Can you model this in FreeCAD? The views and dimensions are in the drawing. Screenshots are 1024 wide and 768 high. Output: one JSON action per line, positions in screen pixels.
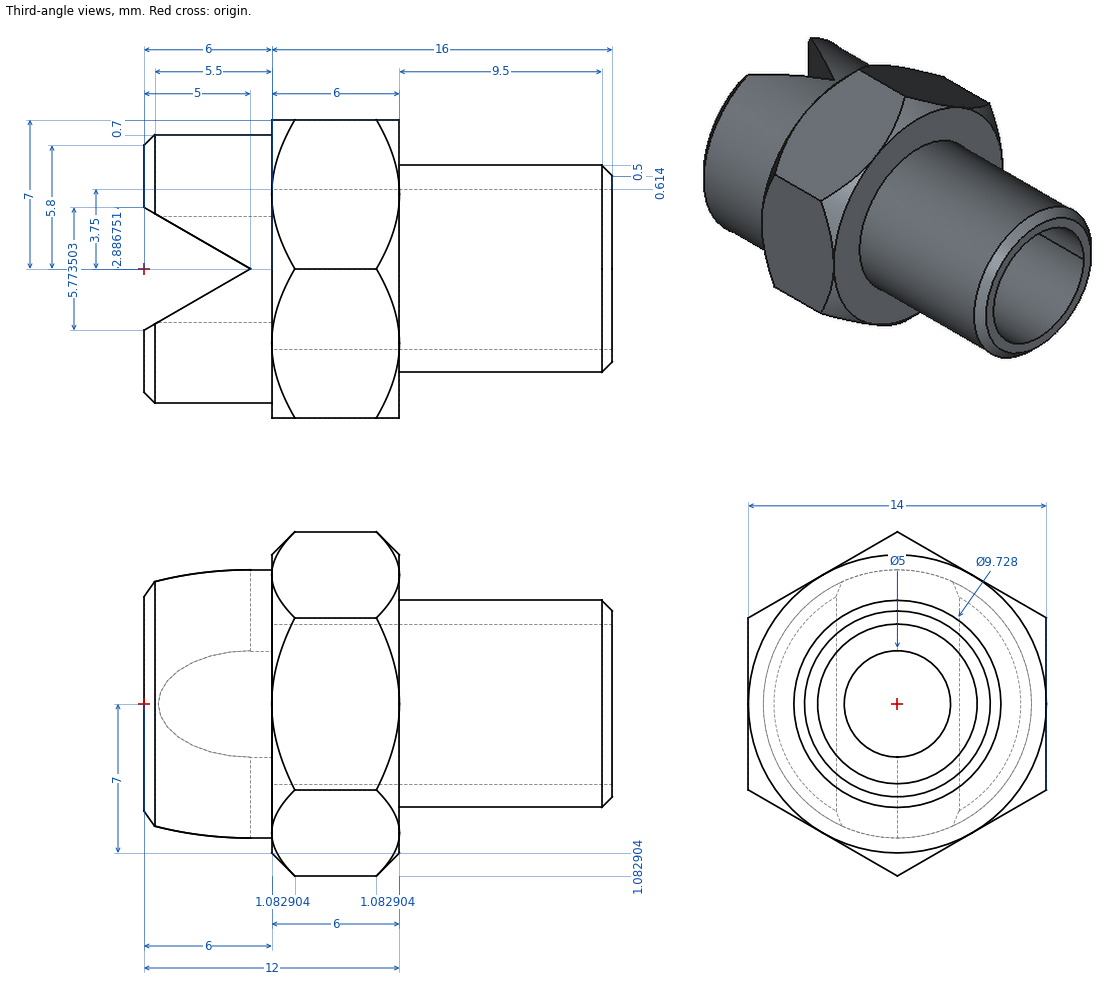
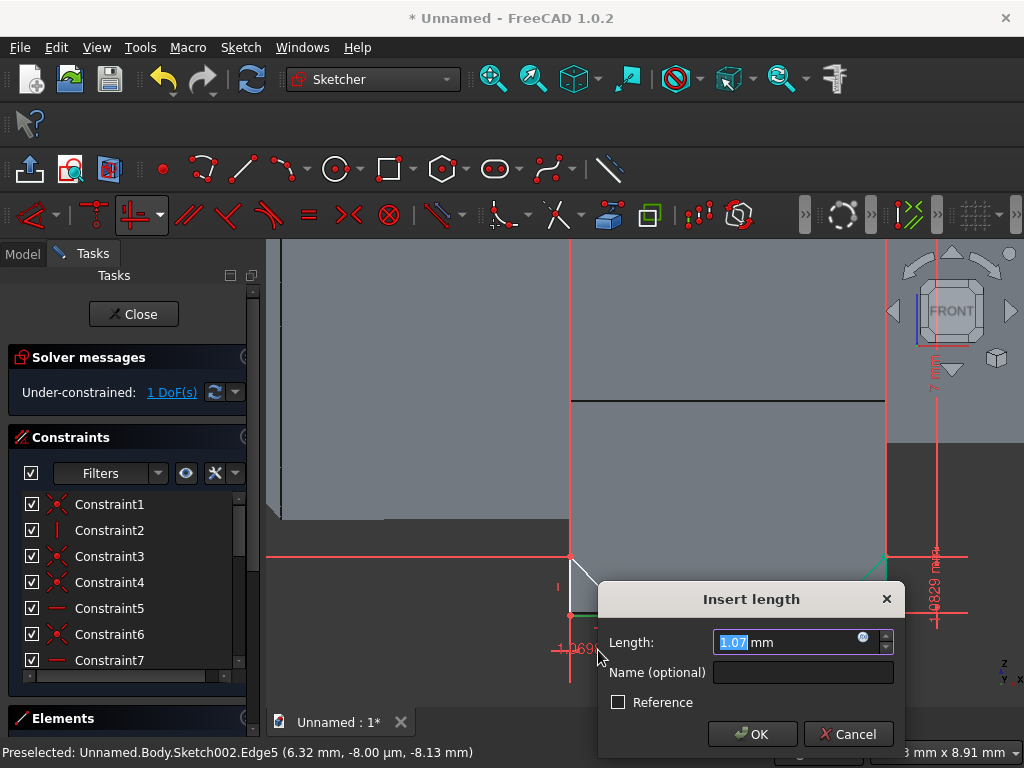
{"action": "type", "text": "1.082904"}
{"action": "key", "text": "Return"}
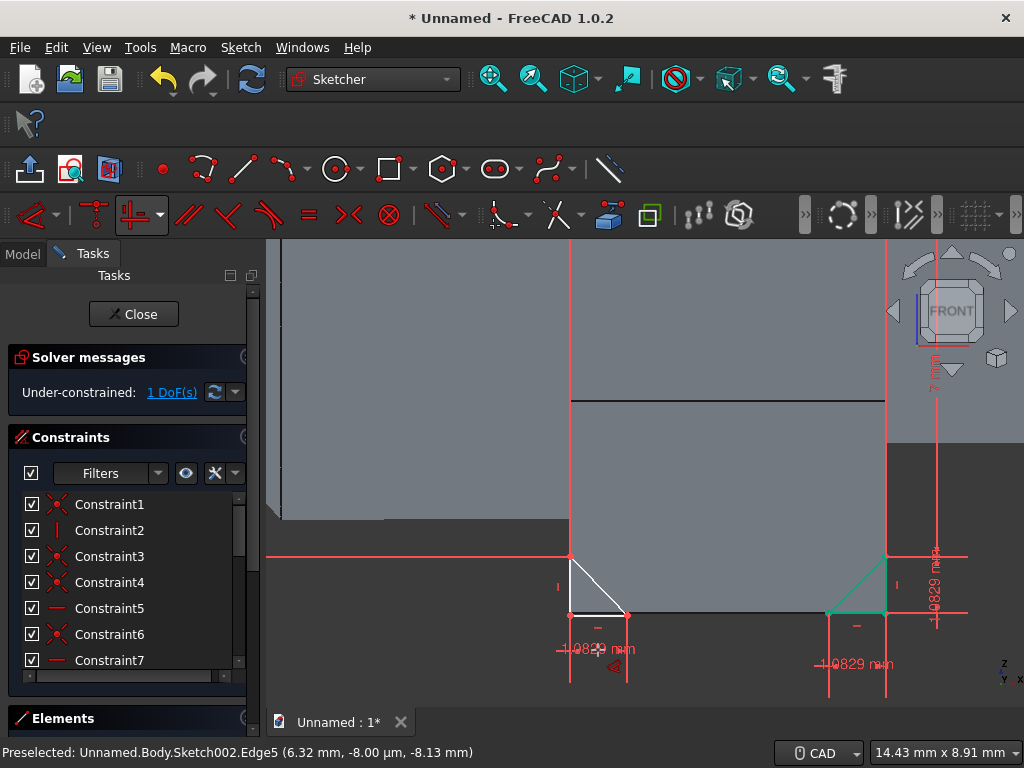
{"action": "left_click", "coordinate": [570, 598]}
{"action": "left_click", "coordinate": [604, 572]}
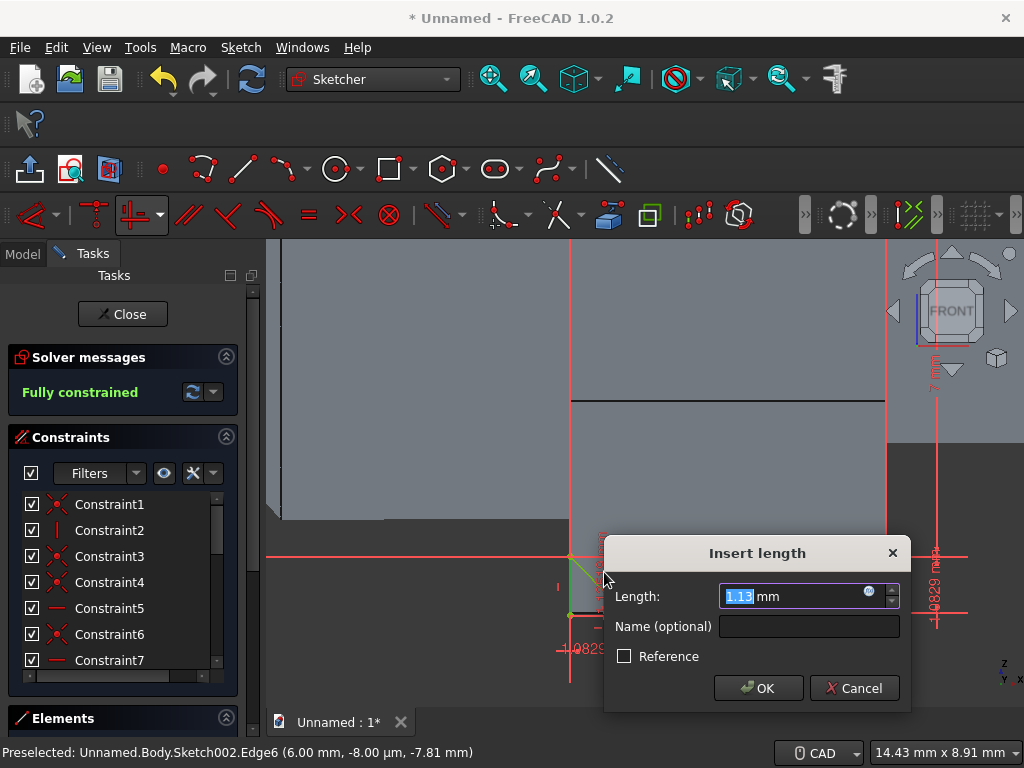
{"action": "type", "text": "1.082904"}
{"action": "key", "text": "Return"}
{"action": "key", "text": "Escape"}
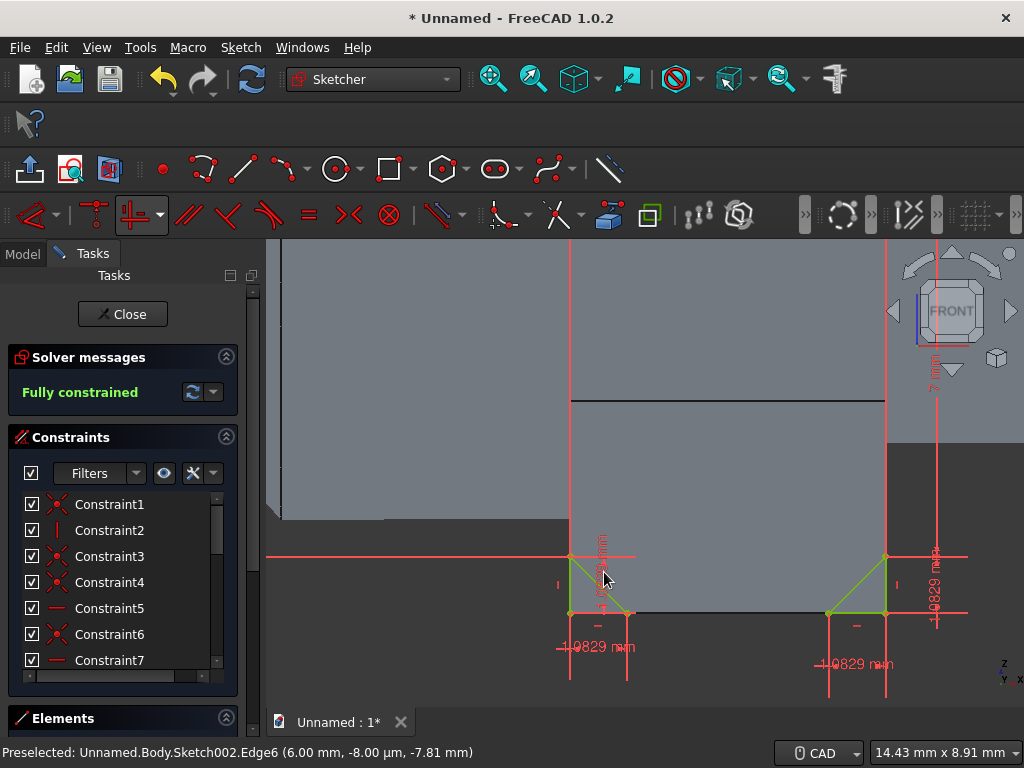
{"action": "left_click", "coordinate": [123, 314]}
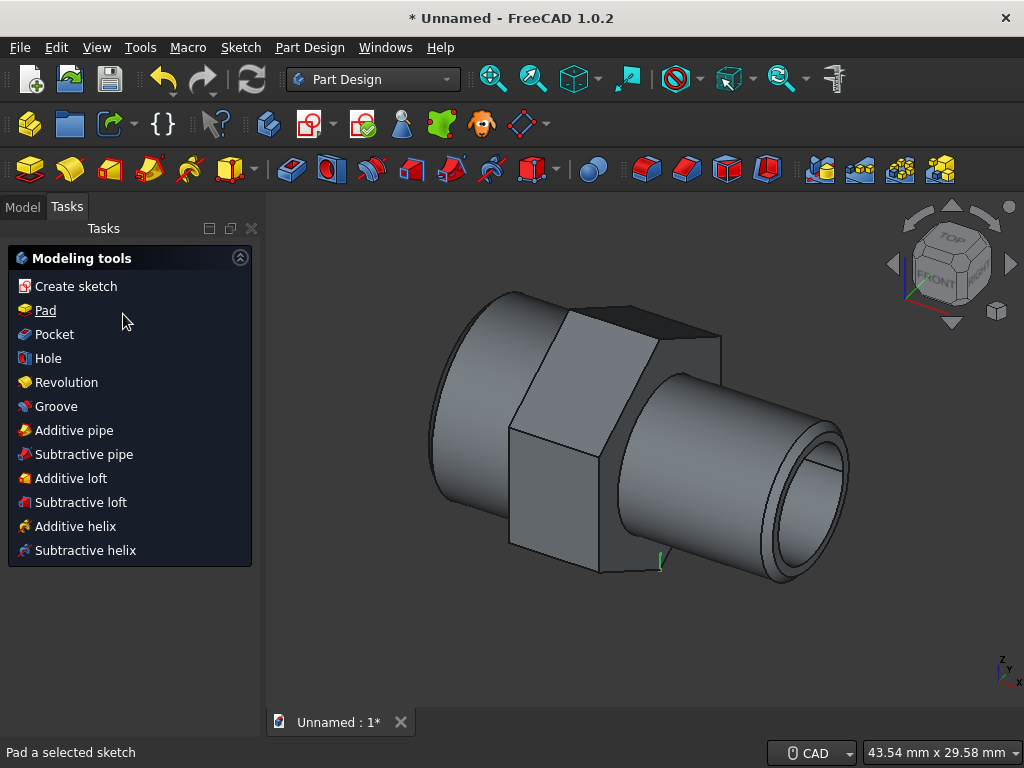
{"action": "left_click", "coordinate": [372, 170]}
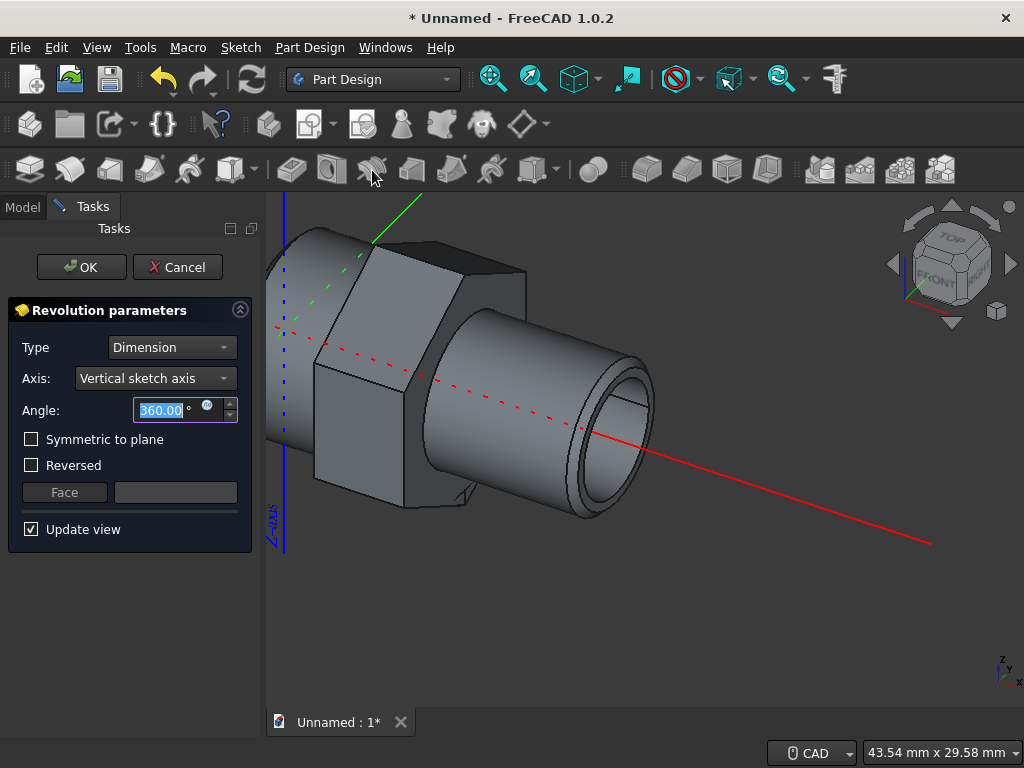
{"action": "left_click", "coordinate": [156, 378]}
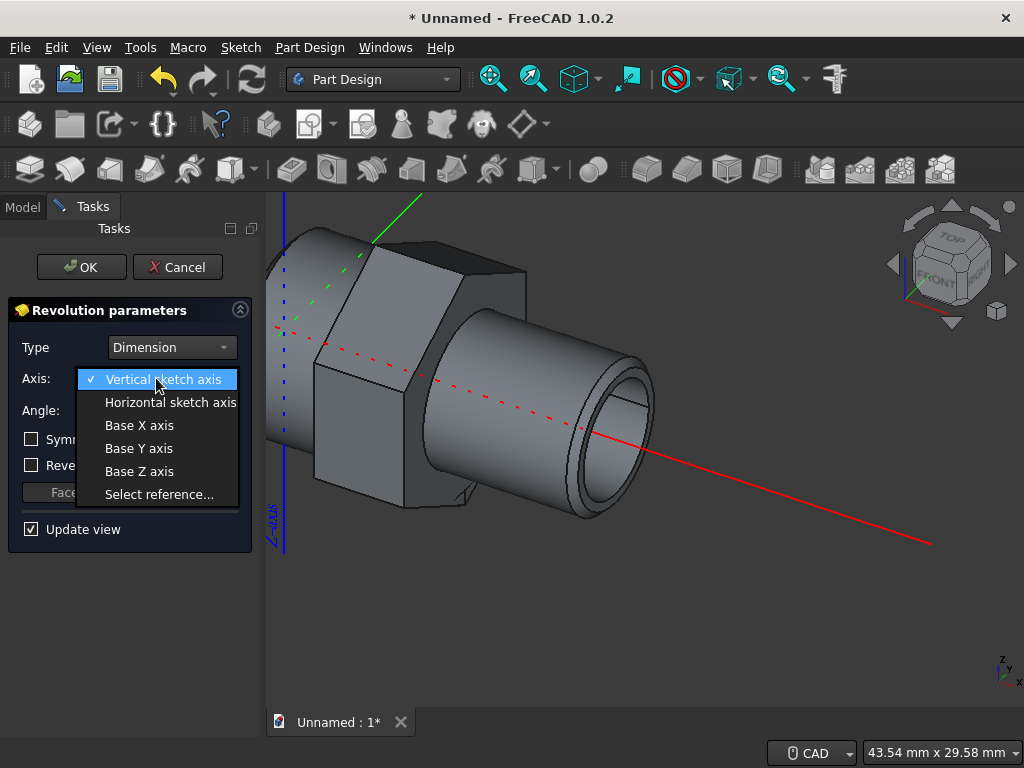
{"action": "left_click", "coordinate": [156, 402]}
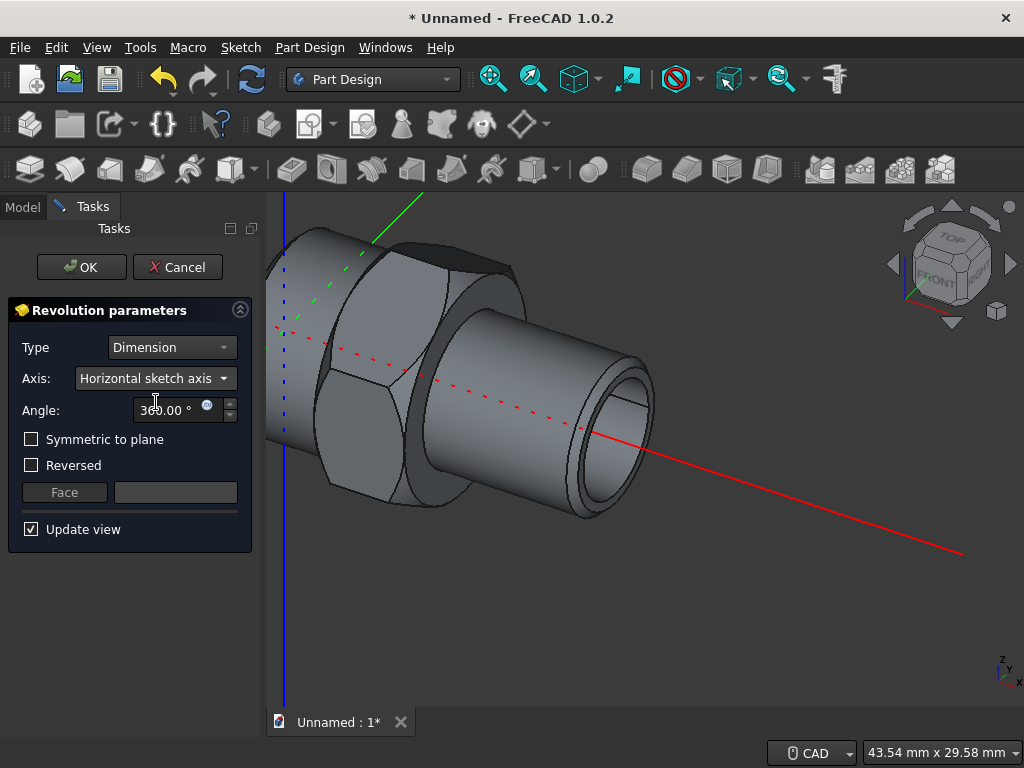
{"action": "left_click", "coordinate": [82, 267]}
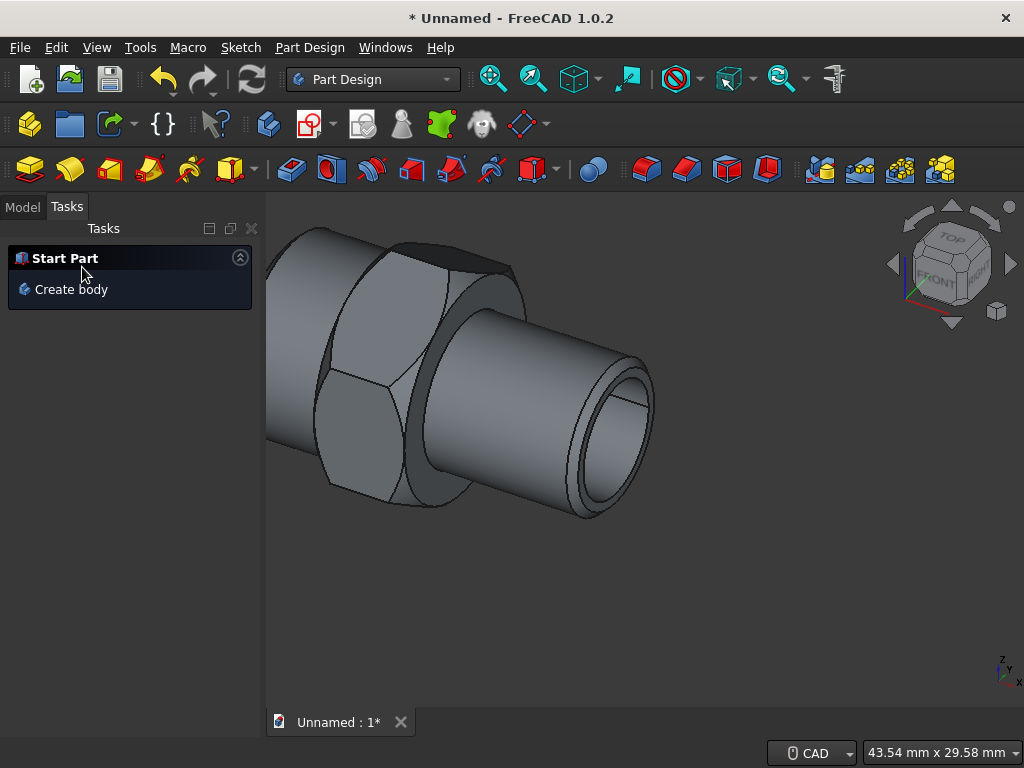
{"action": "left_click", "coordinate": [494, 80]}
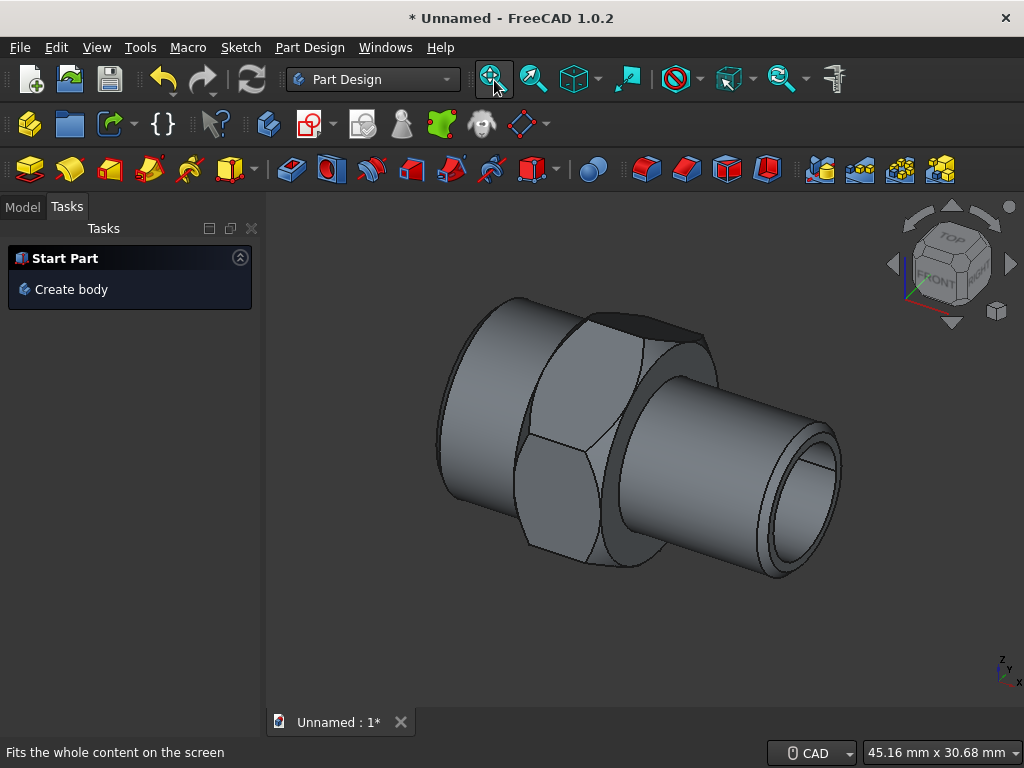
{"action": "left_click", "coordinate": [310, 124]}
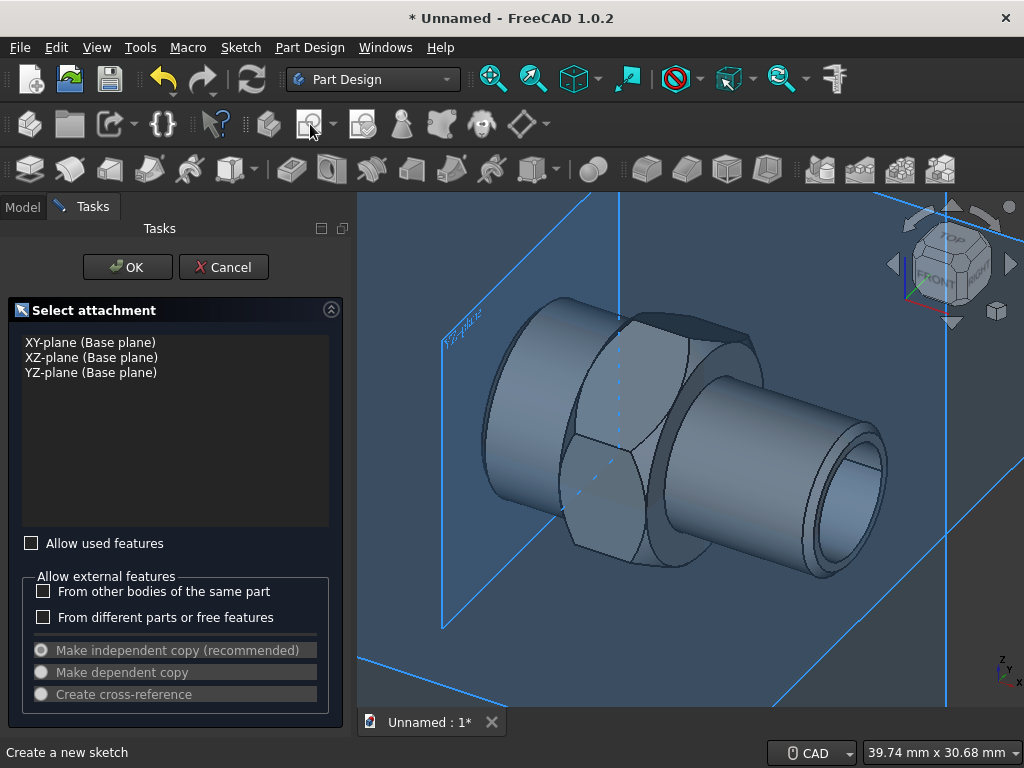
{"action": "left_click", "coordinate": [82, 342]}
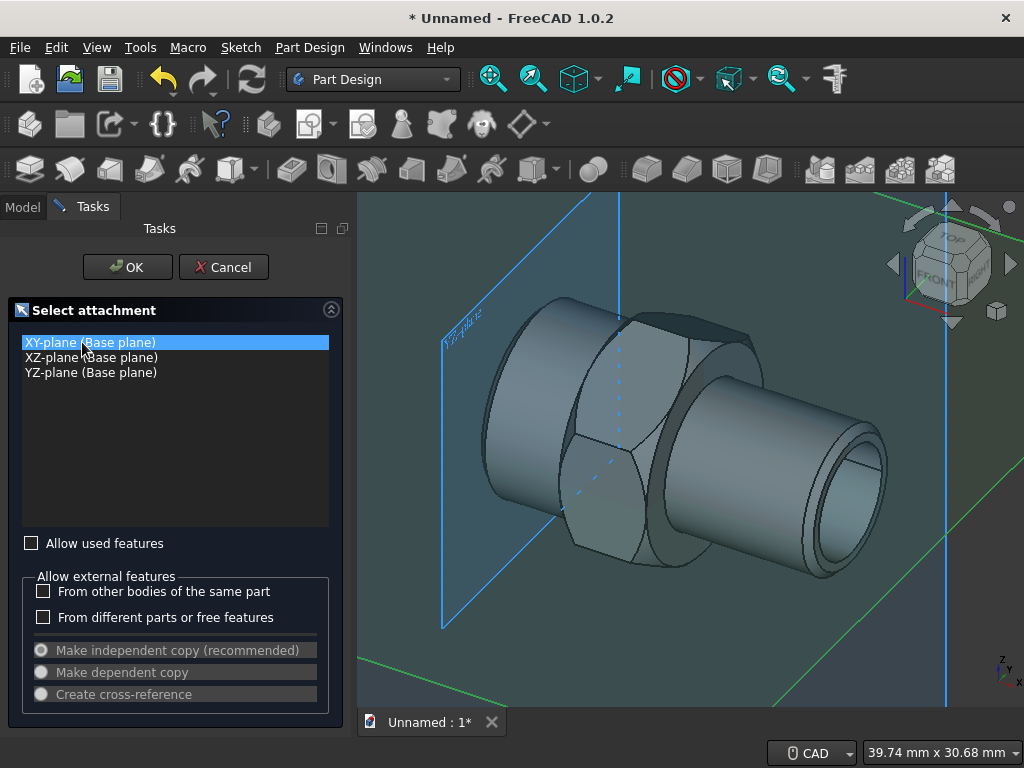
{"action": "left_click", "coordinate": [128, 267]}